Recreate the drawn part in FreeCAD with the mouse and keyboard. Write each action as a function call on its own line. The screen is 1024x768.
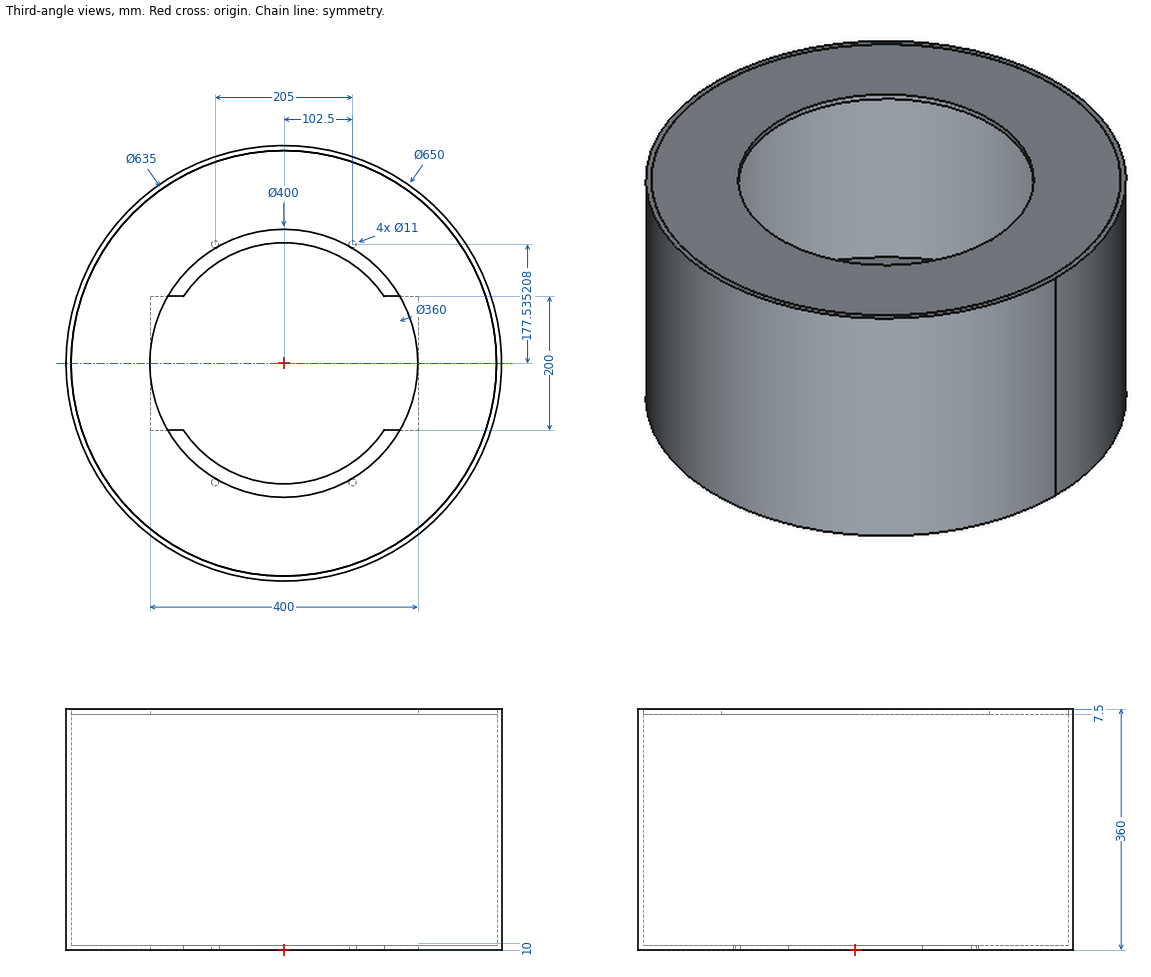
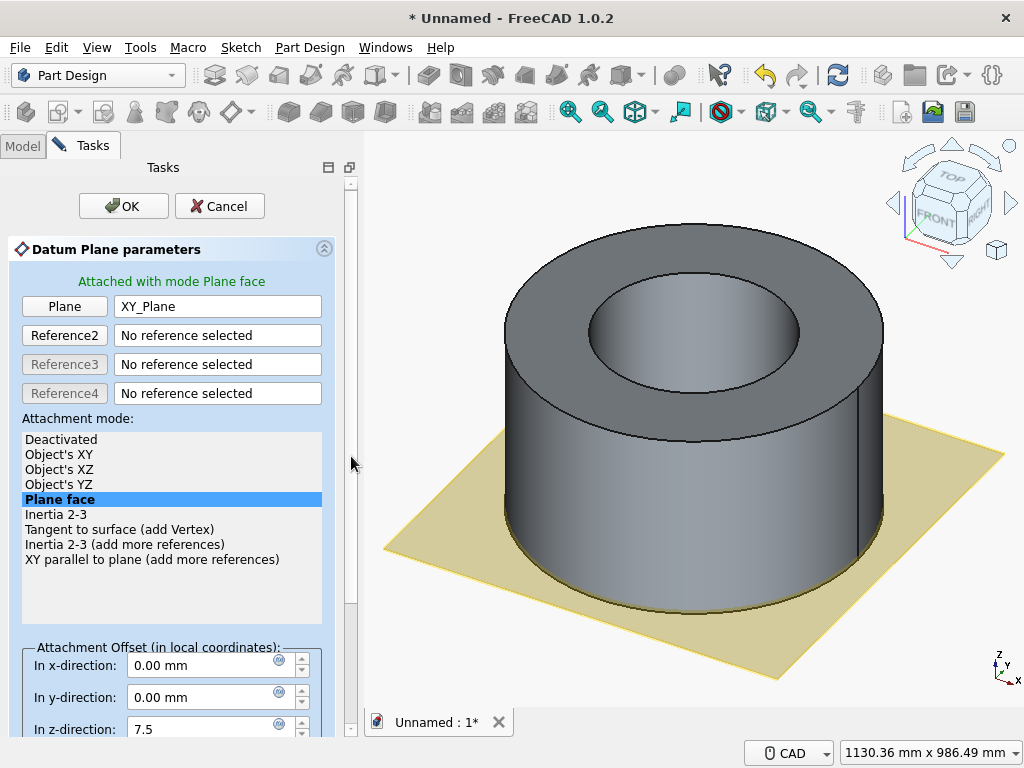
click(124, 206)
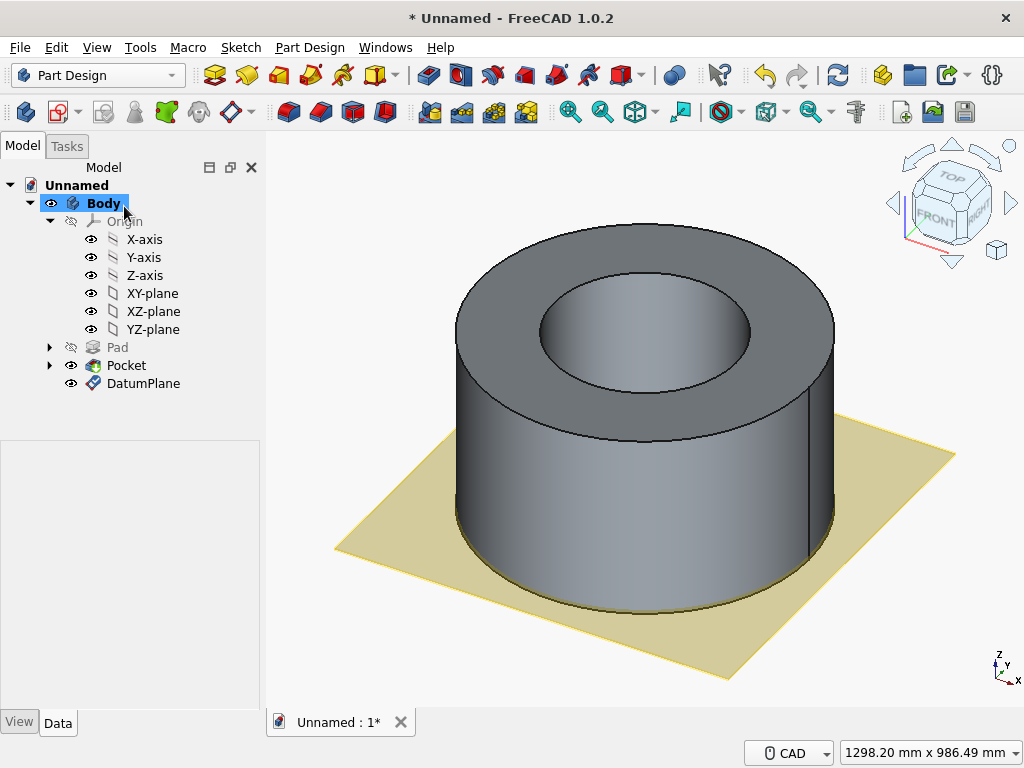
click(116, 383)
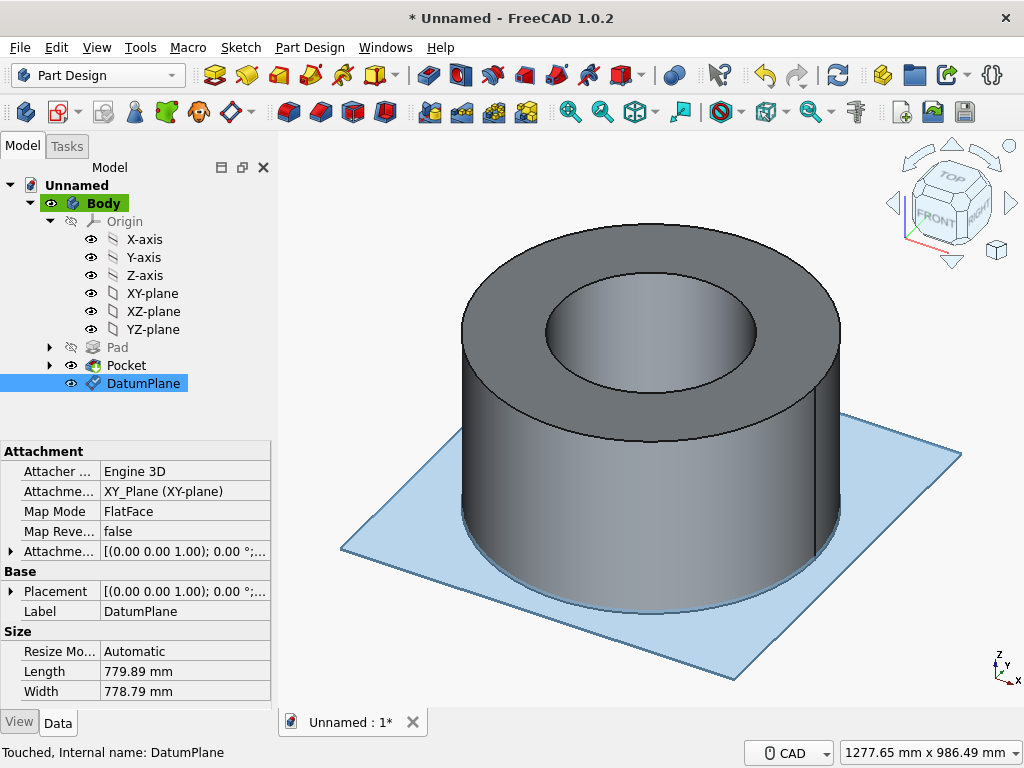
click(58, 112)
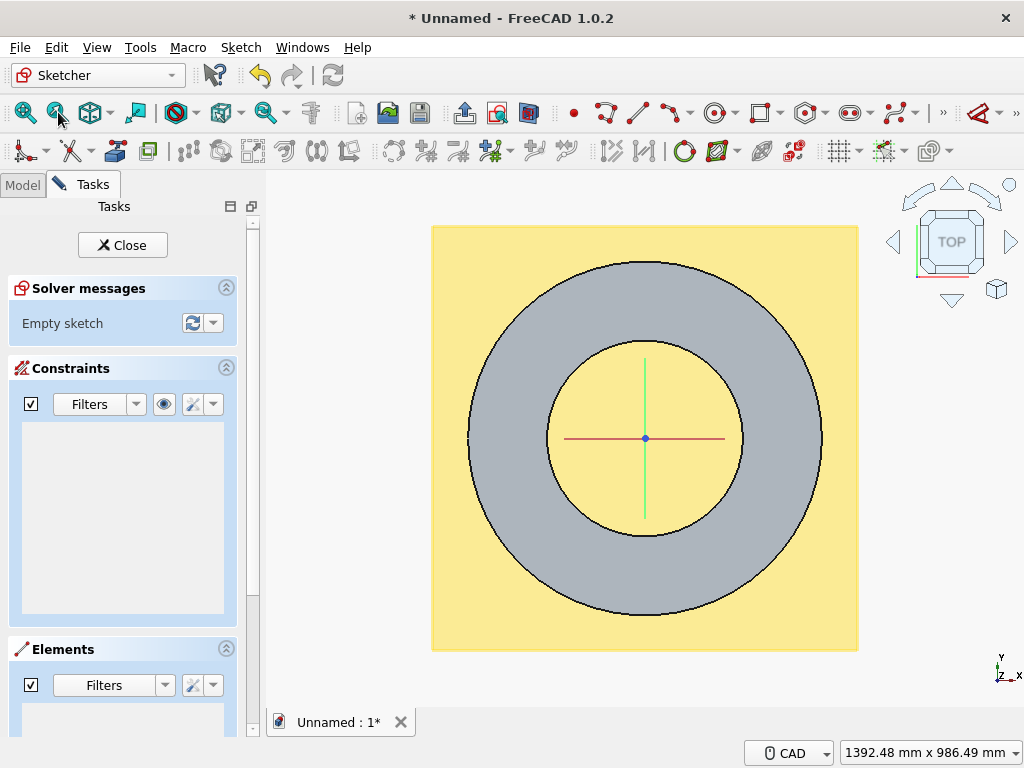
click(530, 114)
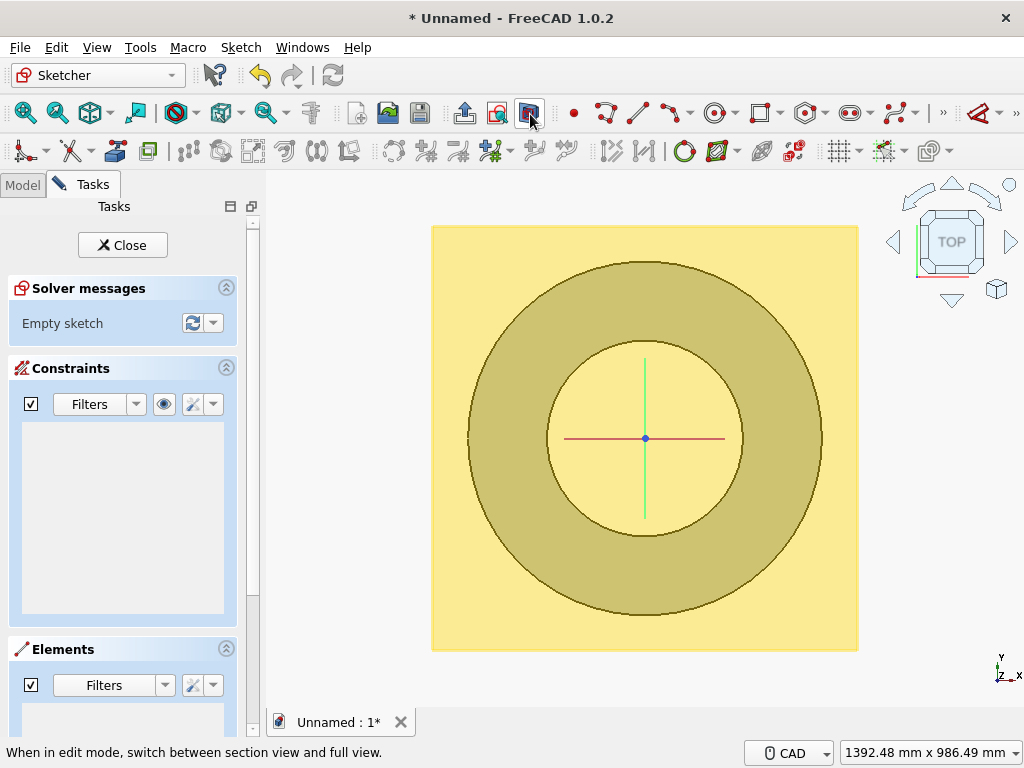
click(716, 114)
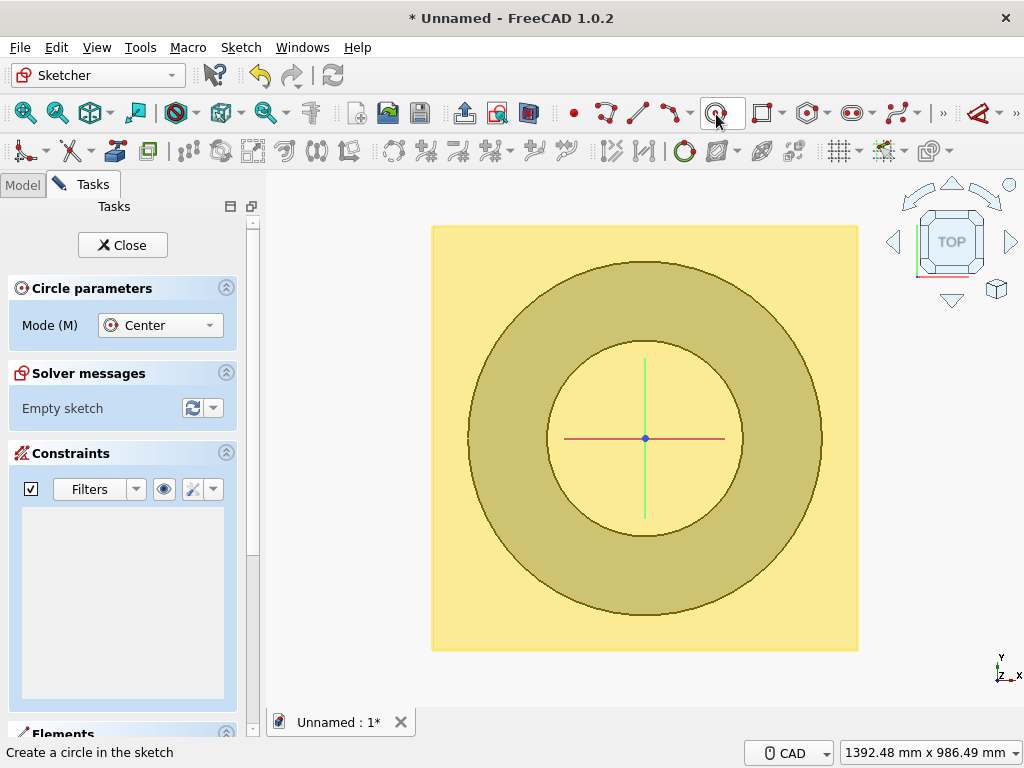
click(645, 438)
click(767, 316)
key(Escape)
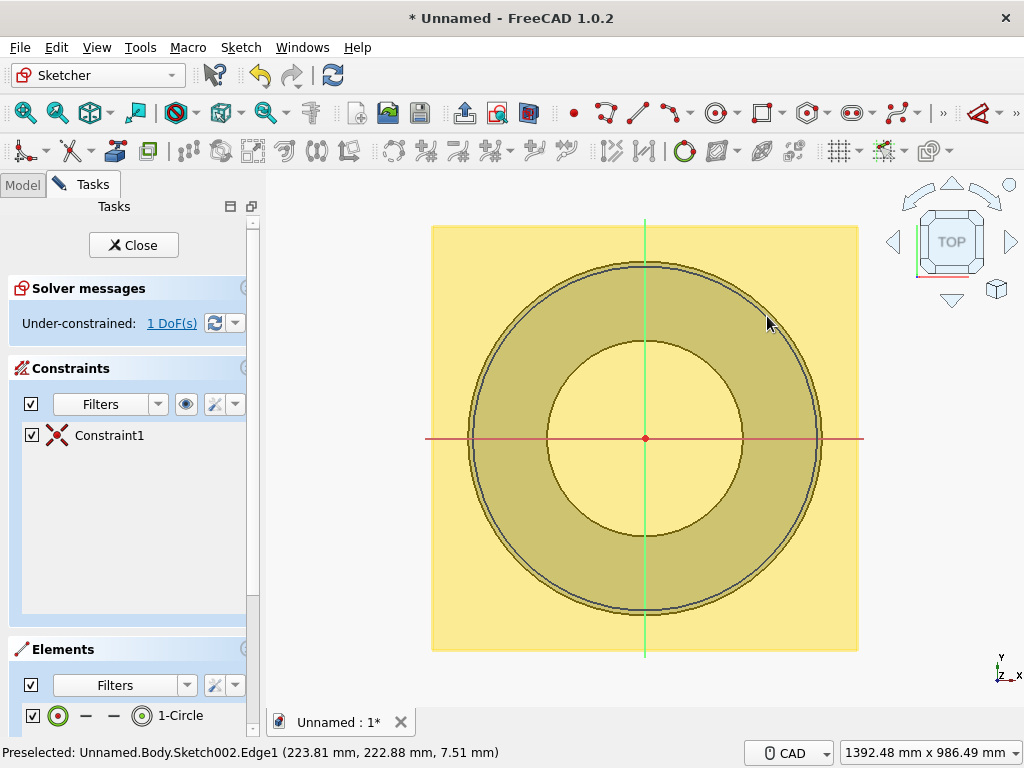
click(978, 114)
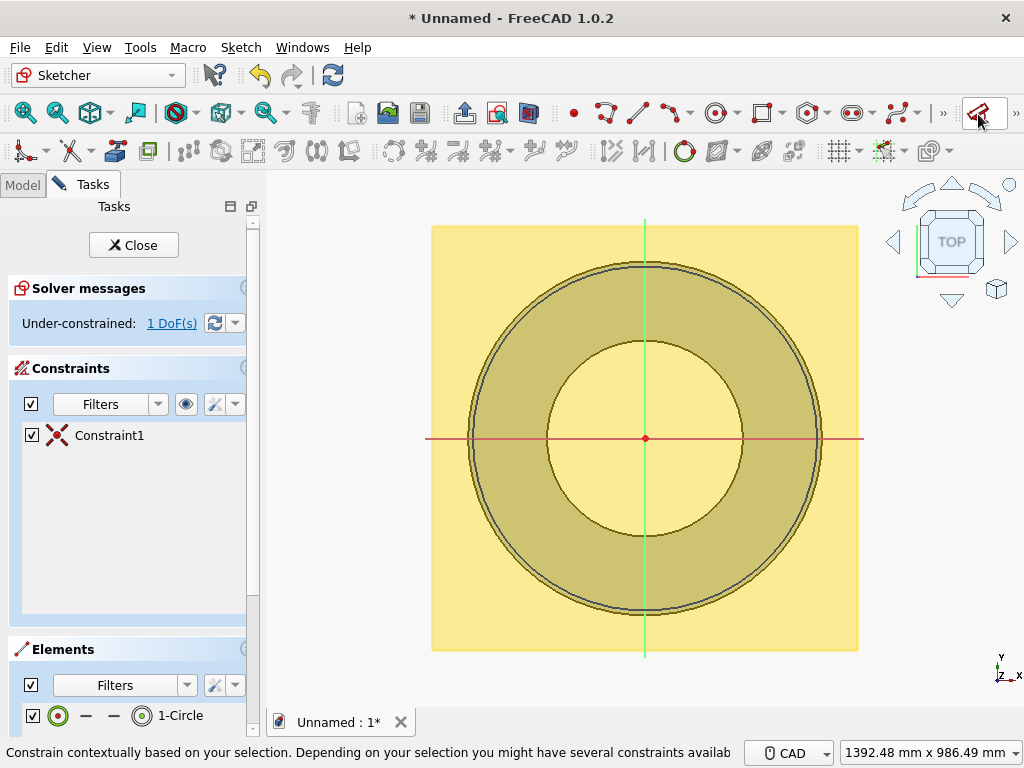
click(766, 316)
click(788, 293)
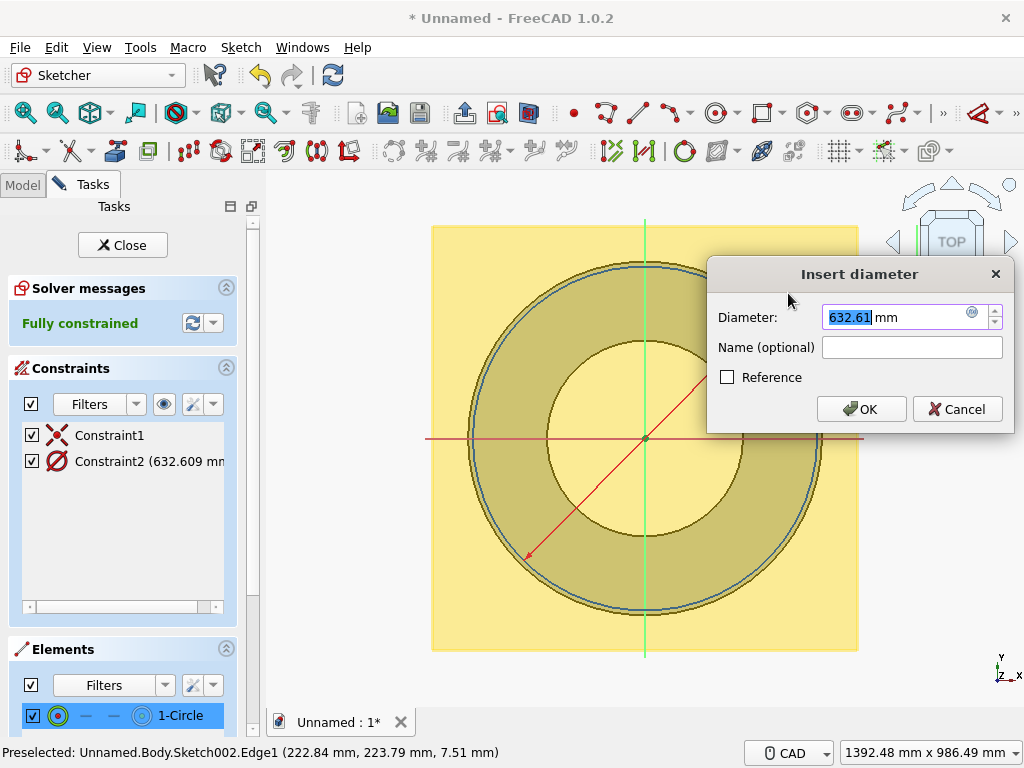
text(635)
key(Return)
key(Escape)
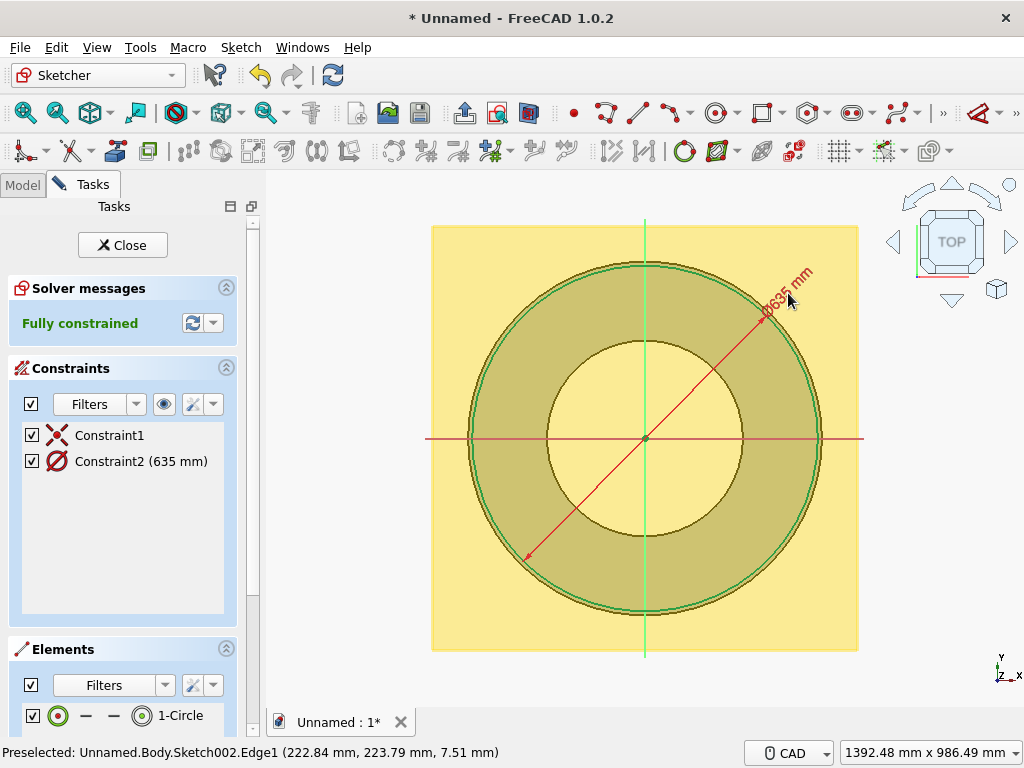
click(123, 245)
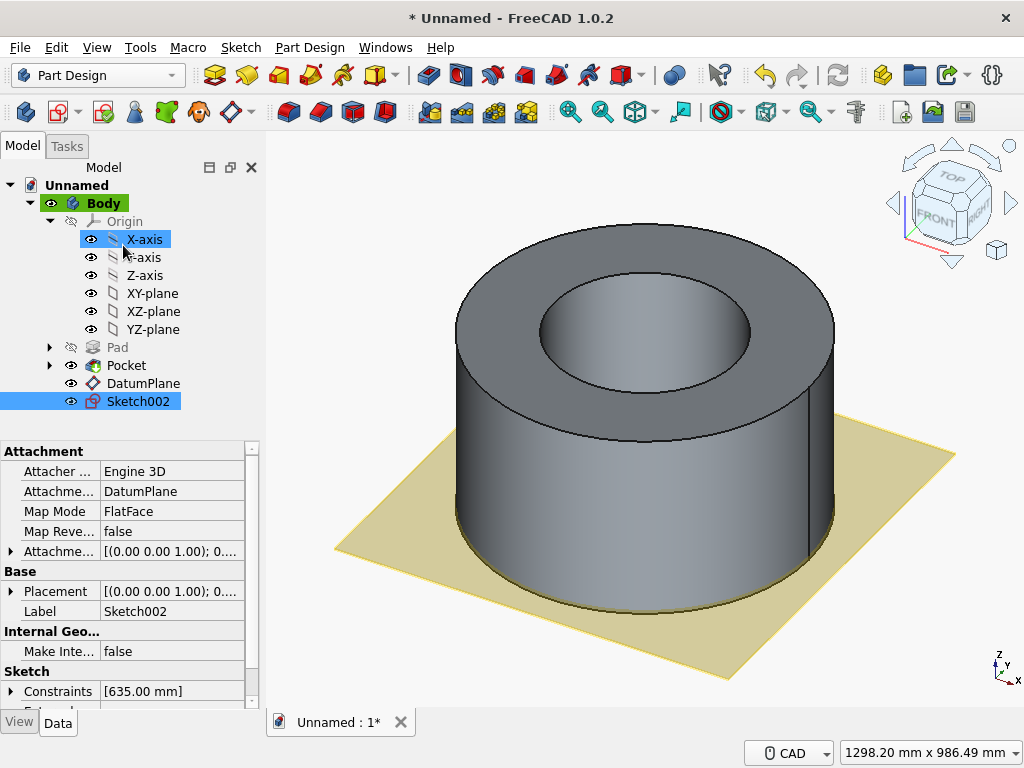
click(430, 76)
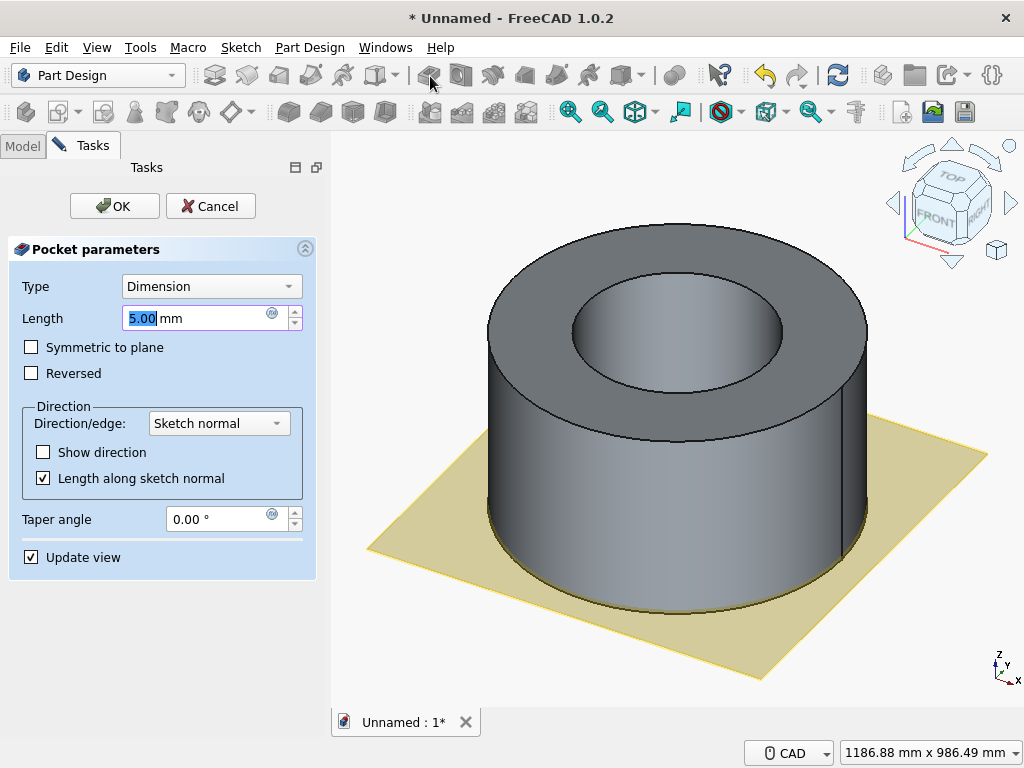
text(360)
key(Tab)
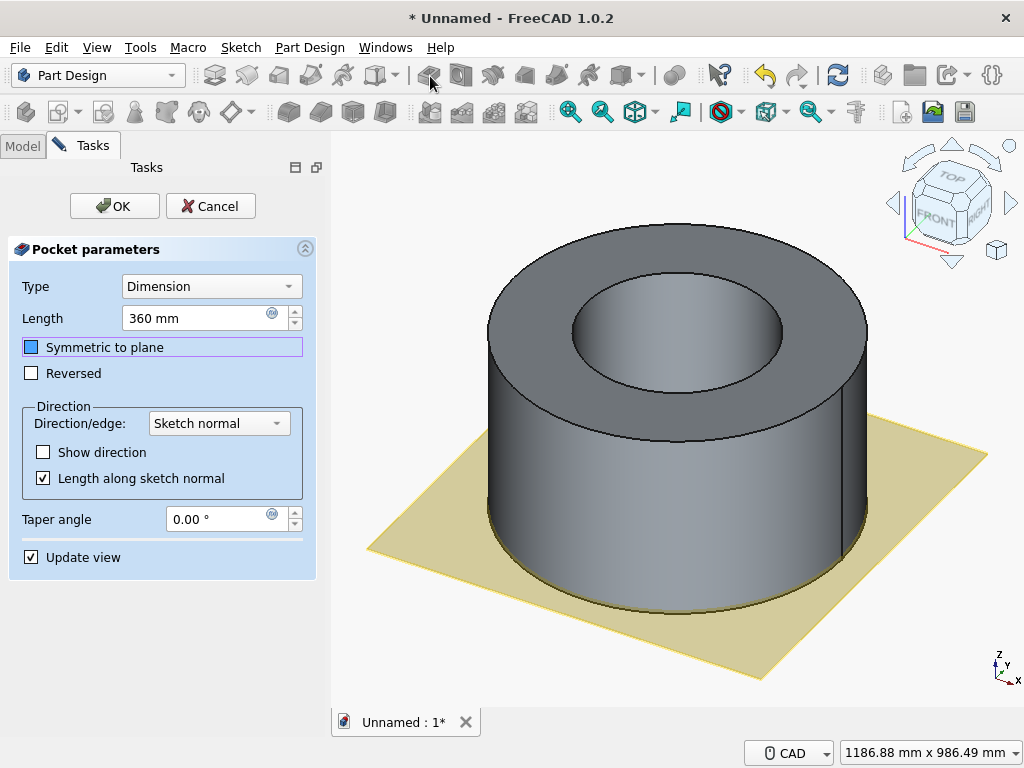
click(30, 373)